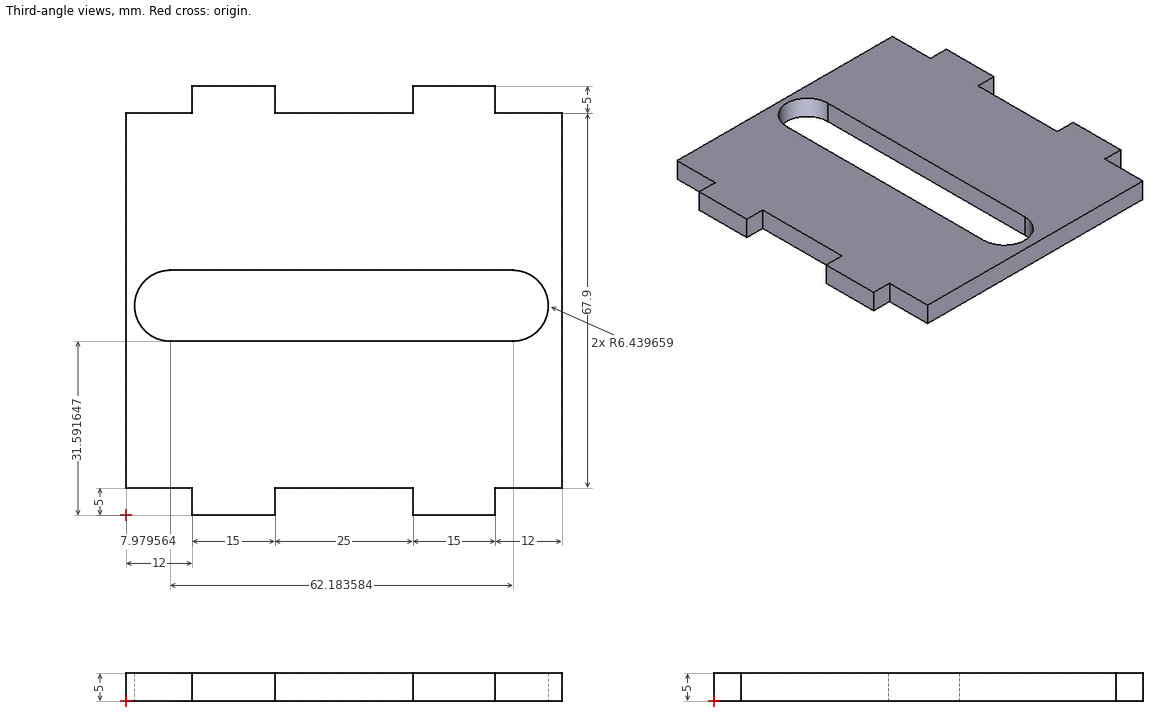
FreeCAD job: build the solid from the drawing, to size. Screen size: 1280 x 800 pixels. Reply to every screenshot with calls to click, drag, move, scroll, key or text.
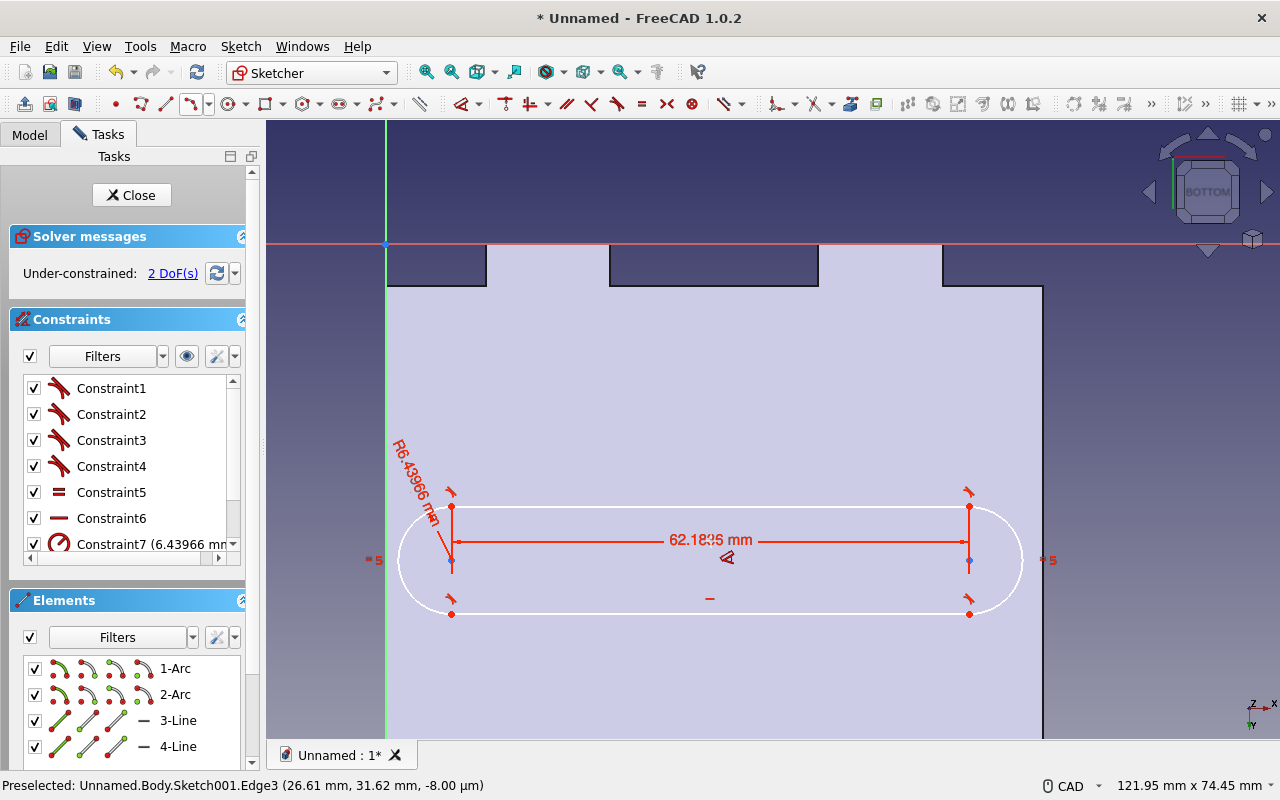
click(452, 507)
click(419, 210)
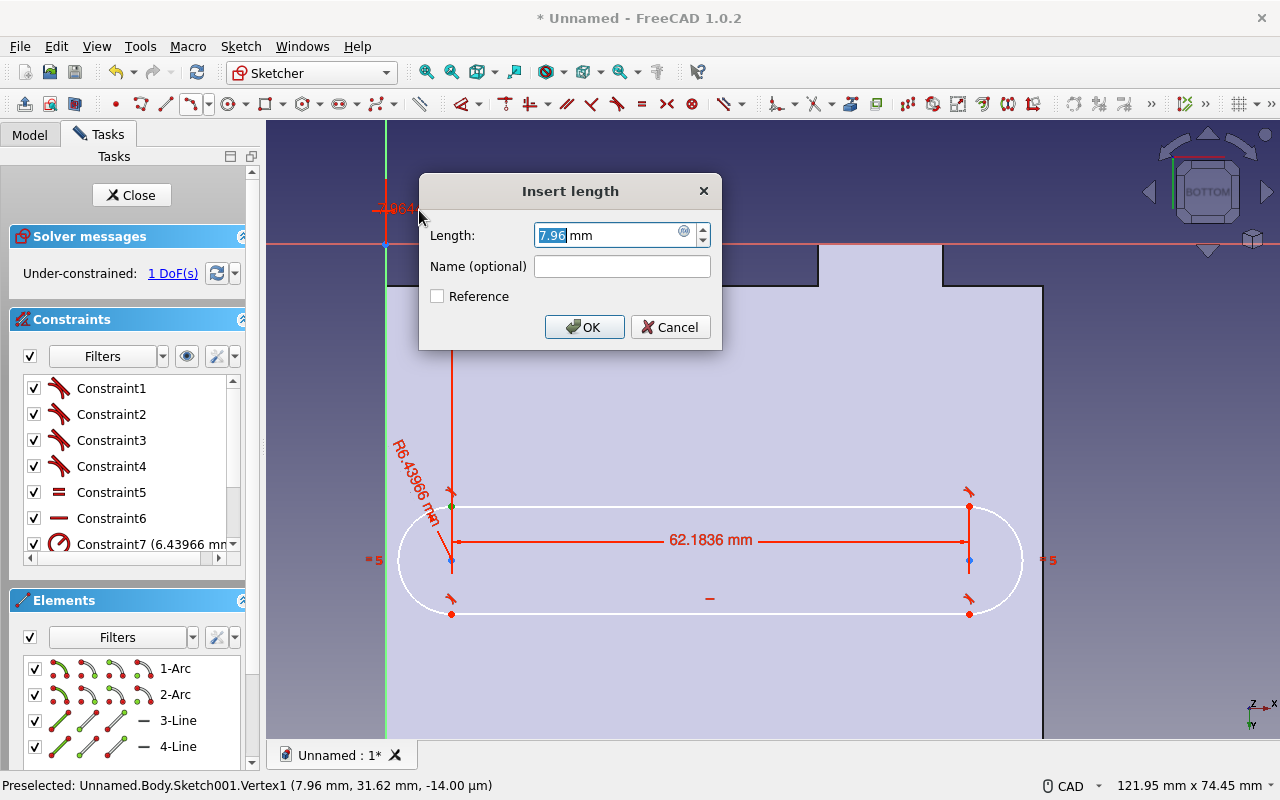
text(7.979564)
key(Return)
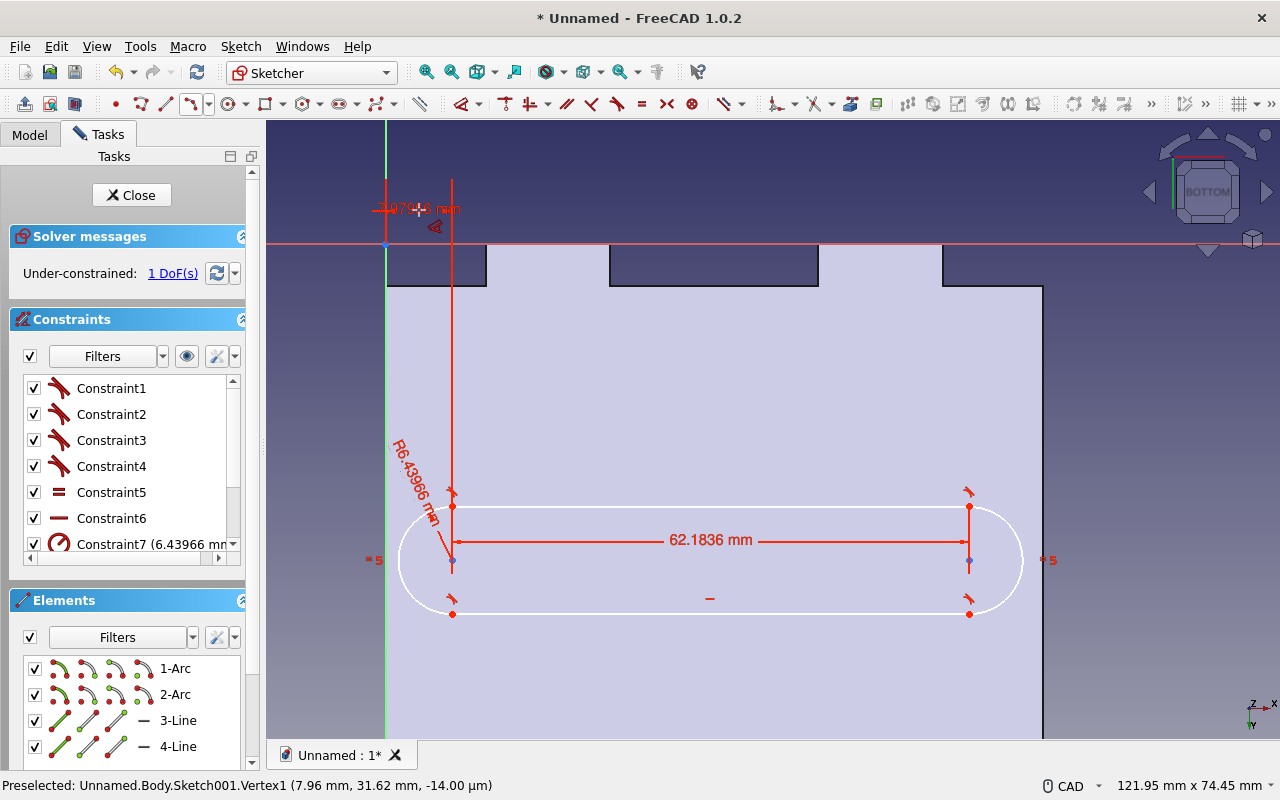
click(452, 507)
click(352, 376)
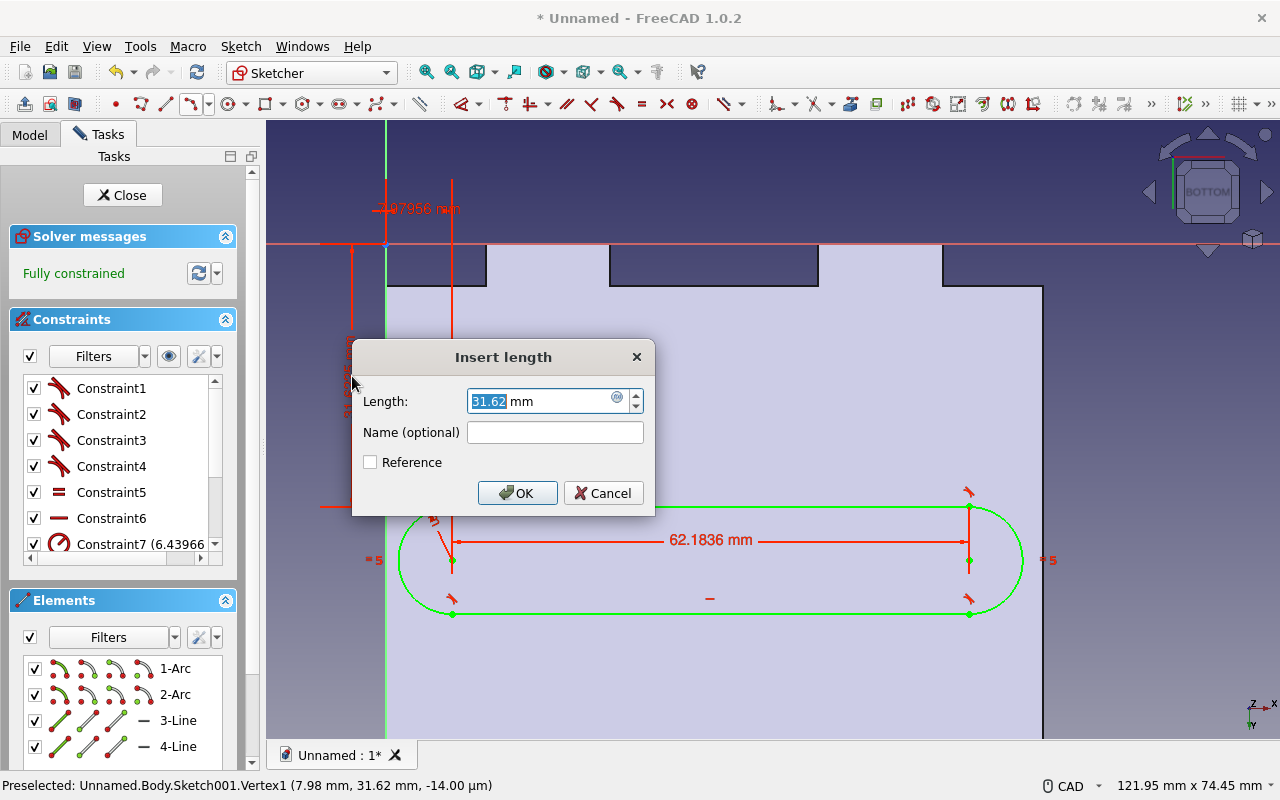
text(31.591647)
key(Return)
key(Escape)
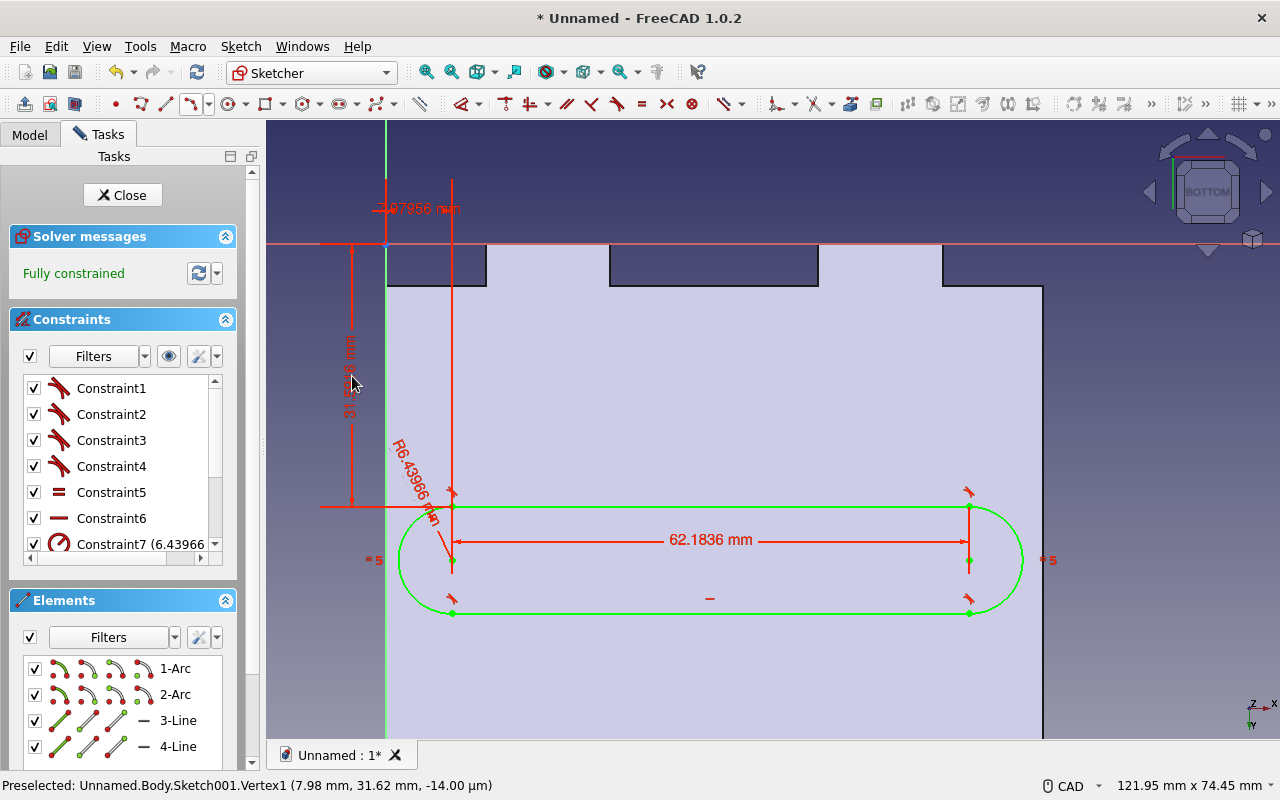
click(123, 195)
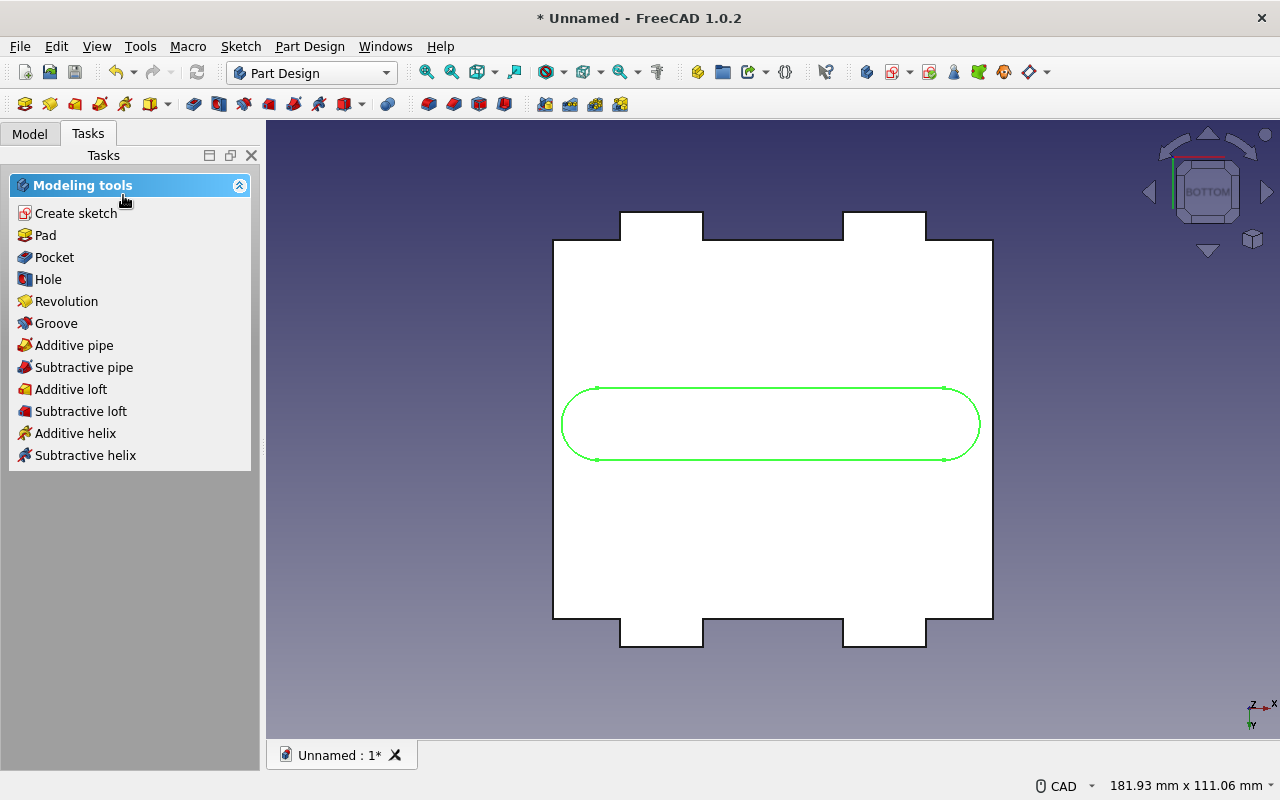
click(194, 104)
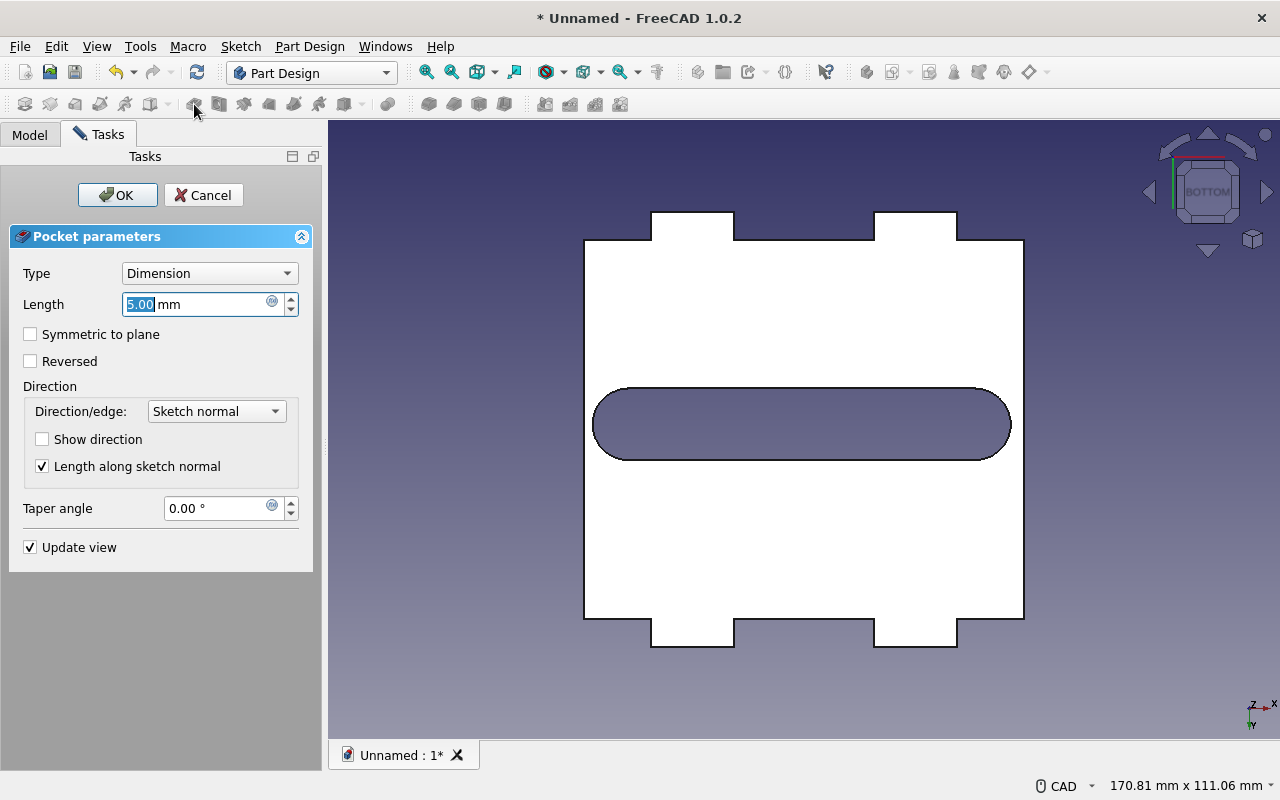
text(5)
key(Tab)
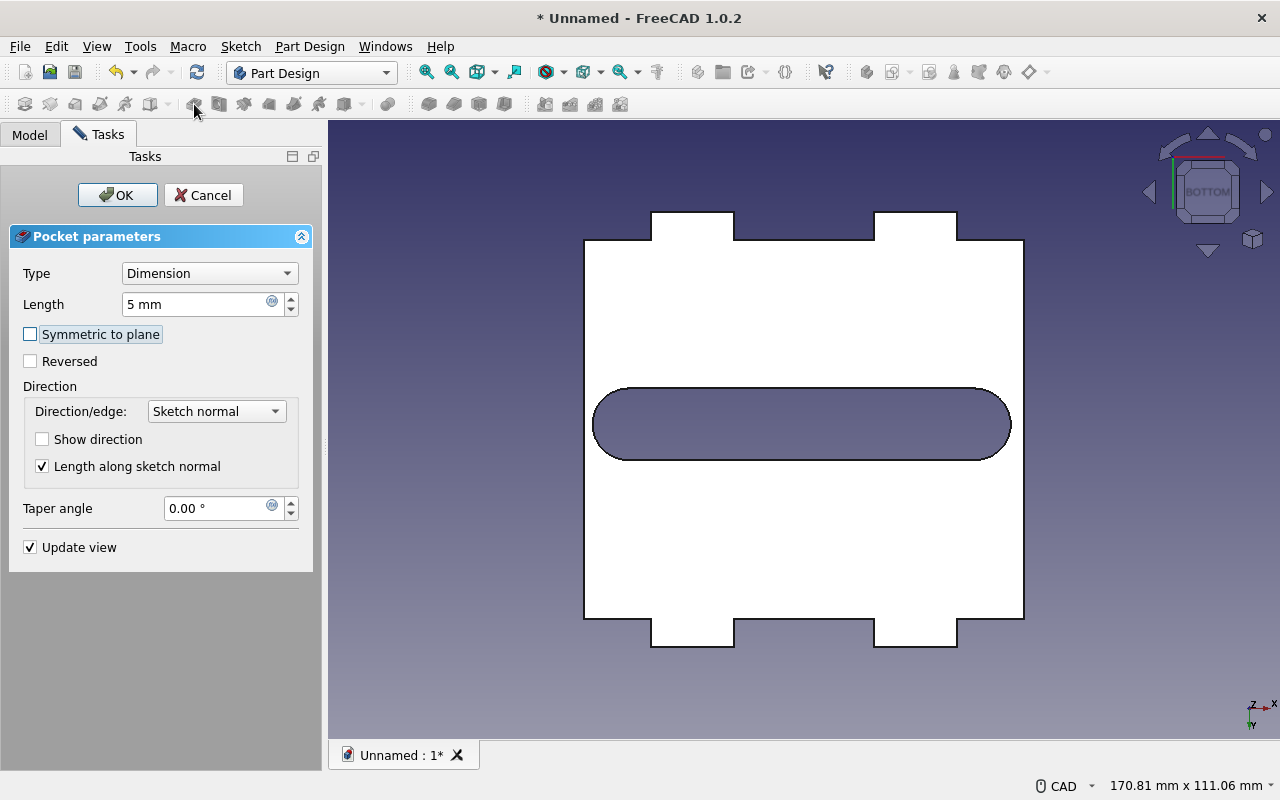
click(118, 195)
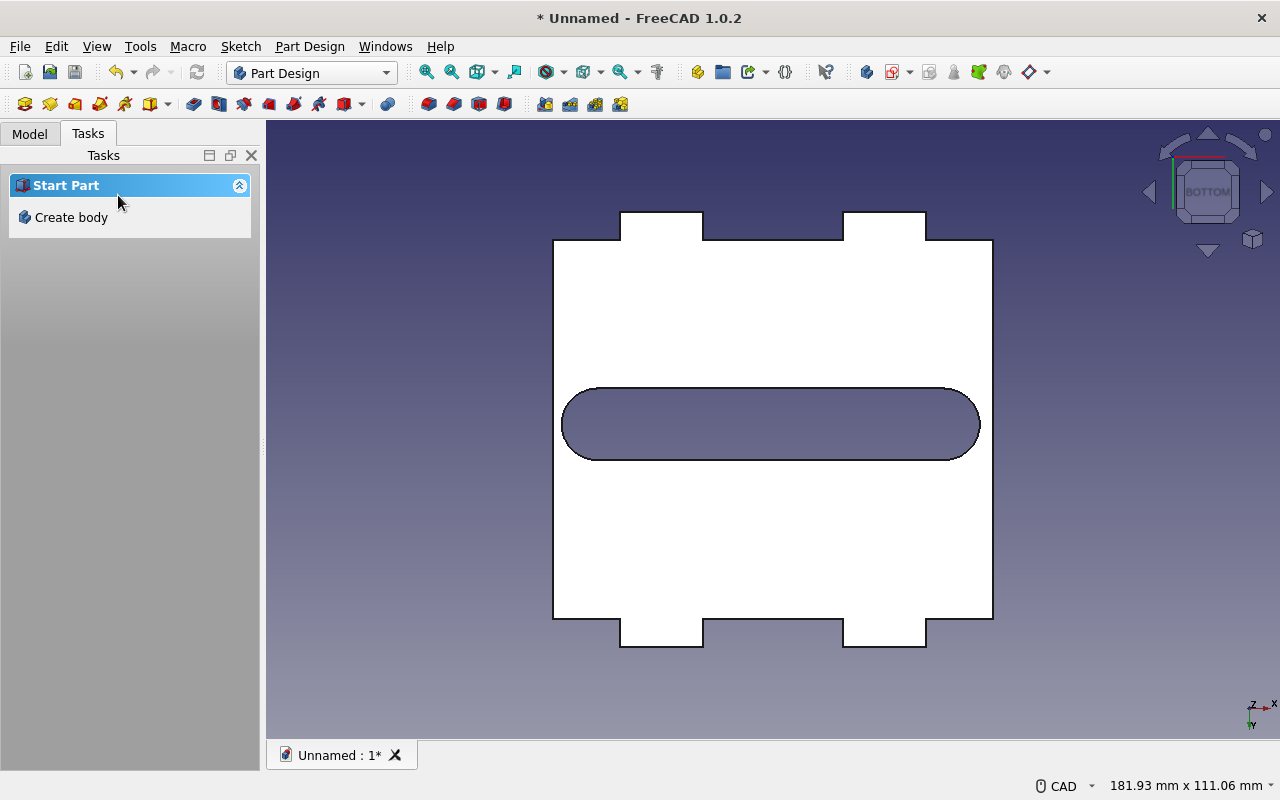
key(0)